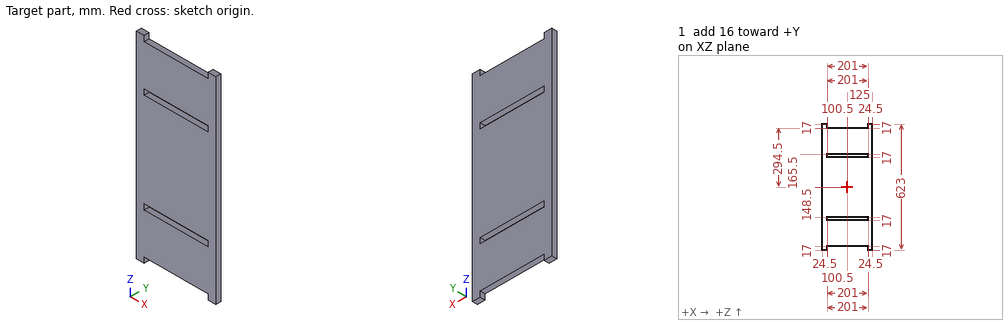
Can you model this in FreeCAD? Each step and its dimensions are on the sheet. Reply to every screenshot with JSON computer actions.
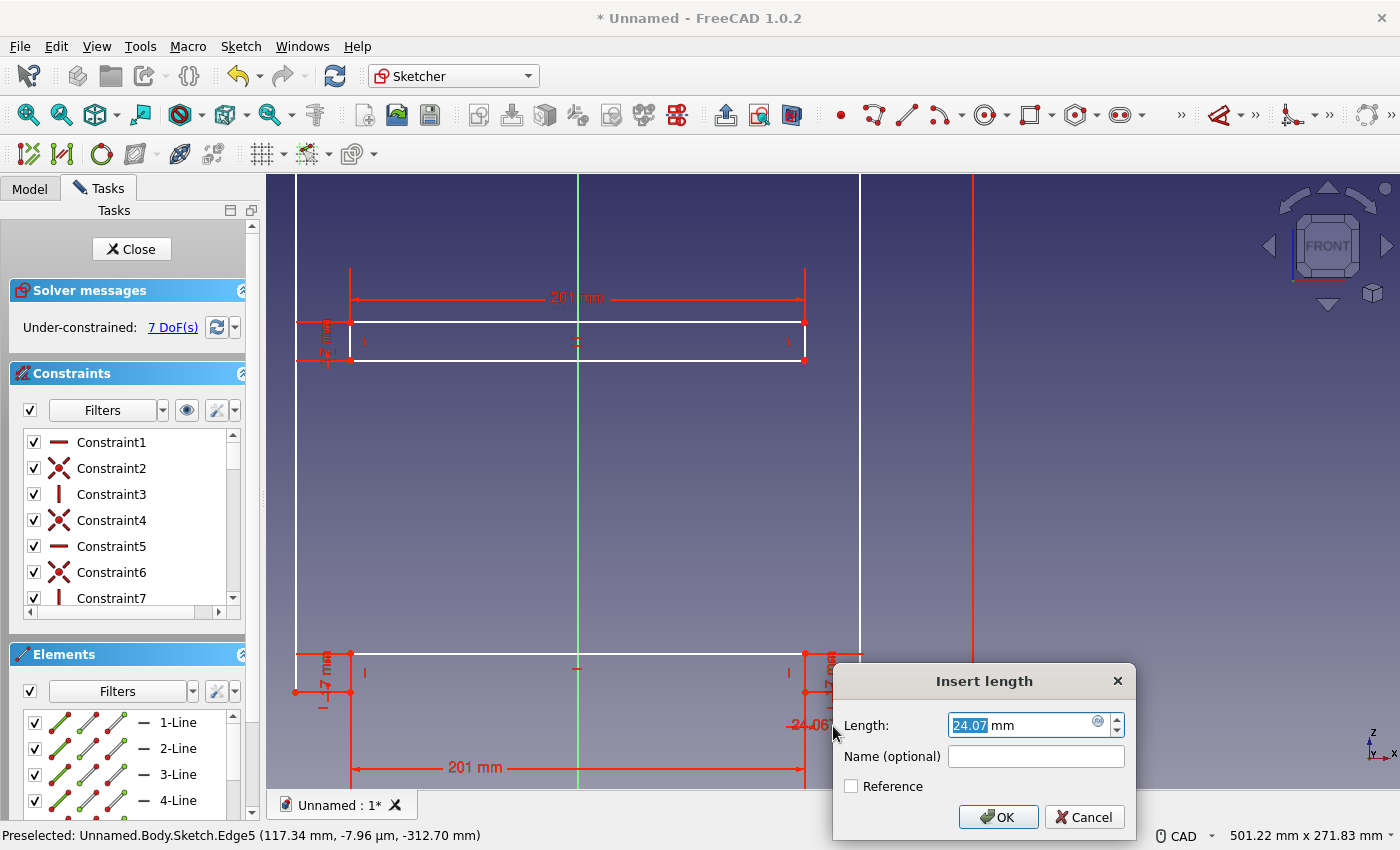
{"action": "type", "text": "24.5"}
{"action": "key", "text": "Return"}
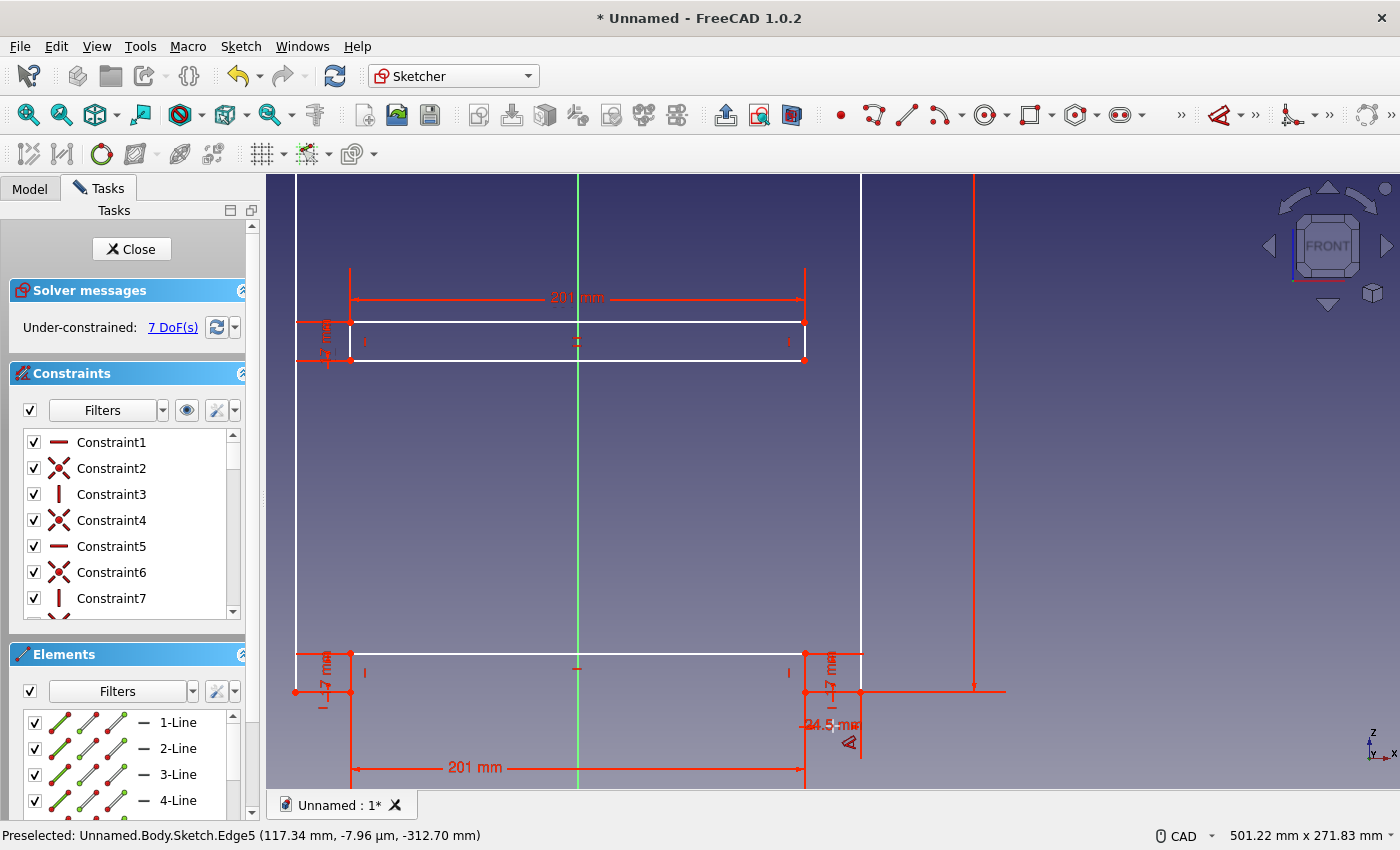
{"action": "left_click", "coordinate": [334, 692]}
{"action": "left_click", "coordinate": [323, 726]}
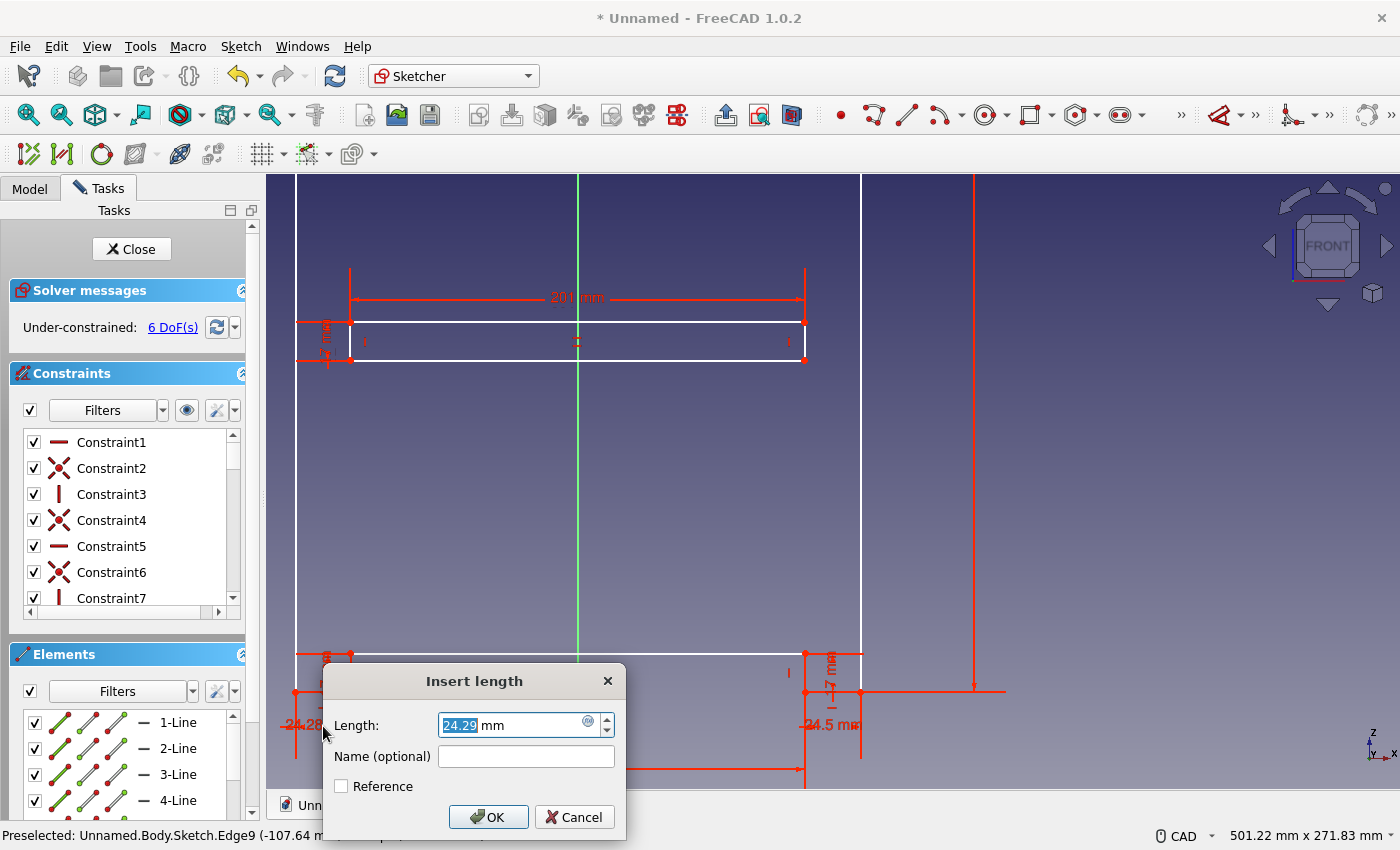
{"action": "type", "text": "24.5"}
{"action": "key", "text": "Return"}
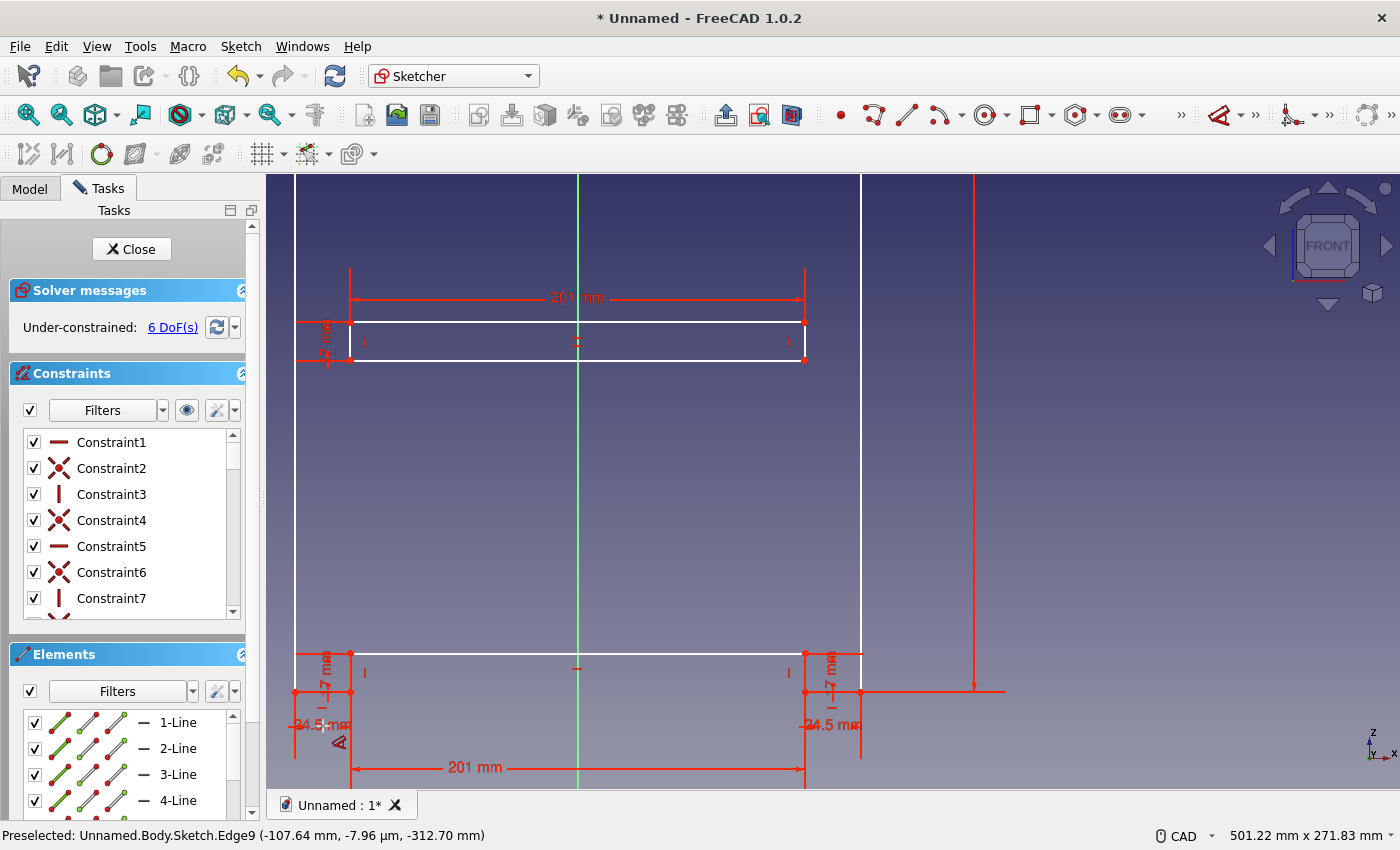
{"action": "scroll", "coordinate": [845, 696], "scroll_direction": "down", "scroll_amount": 6}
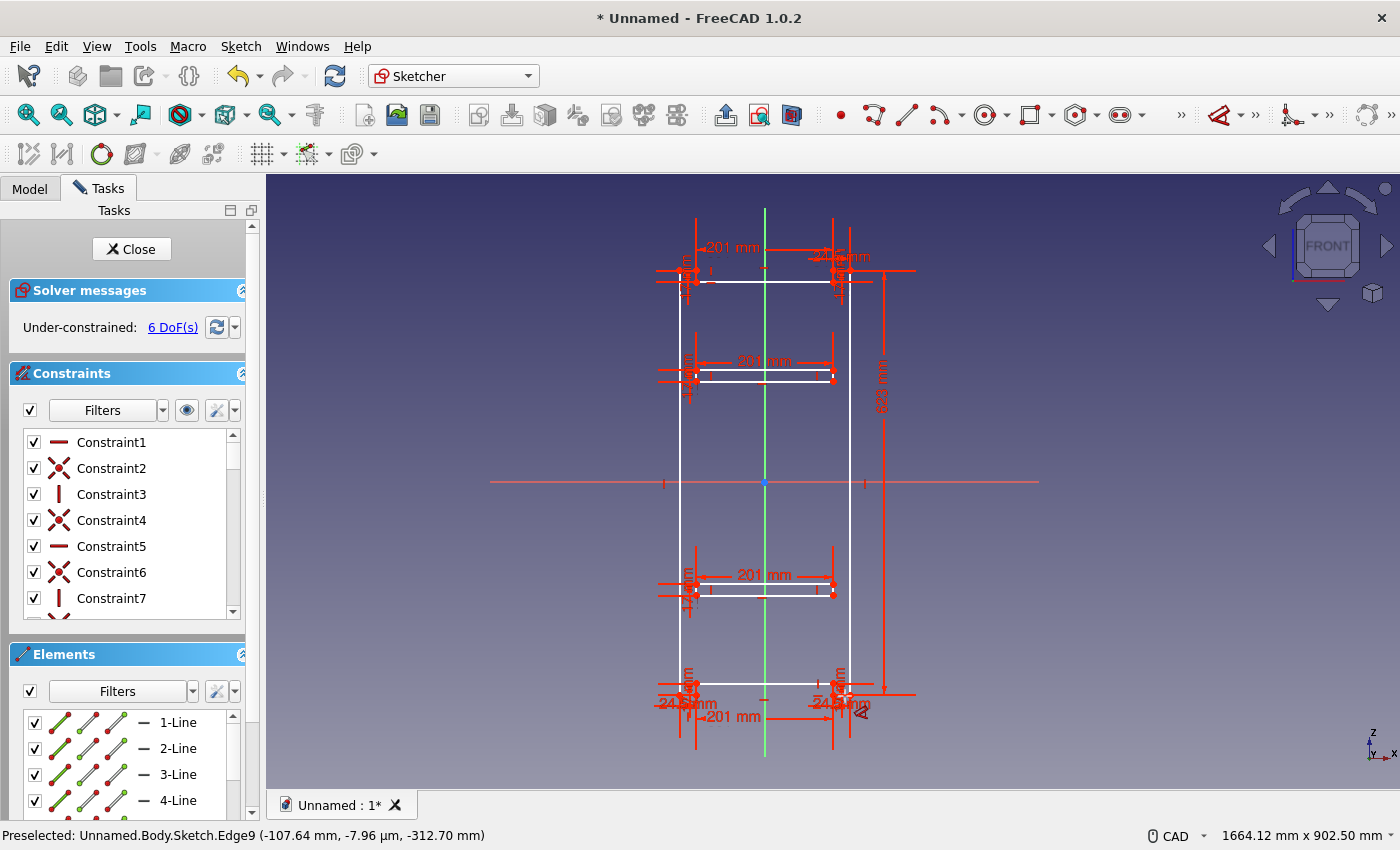
{"action": "left_click", "coordinate": [850, 271]}
{"action": "left_click", "coordinate": [807, 237]}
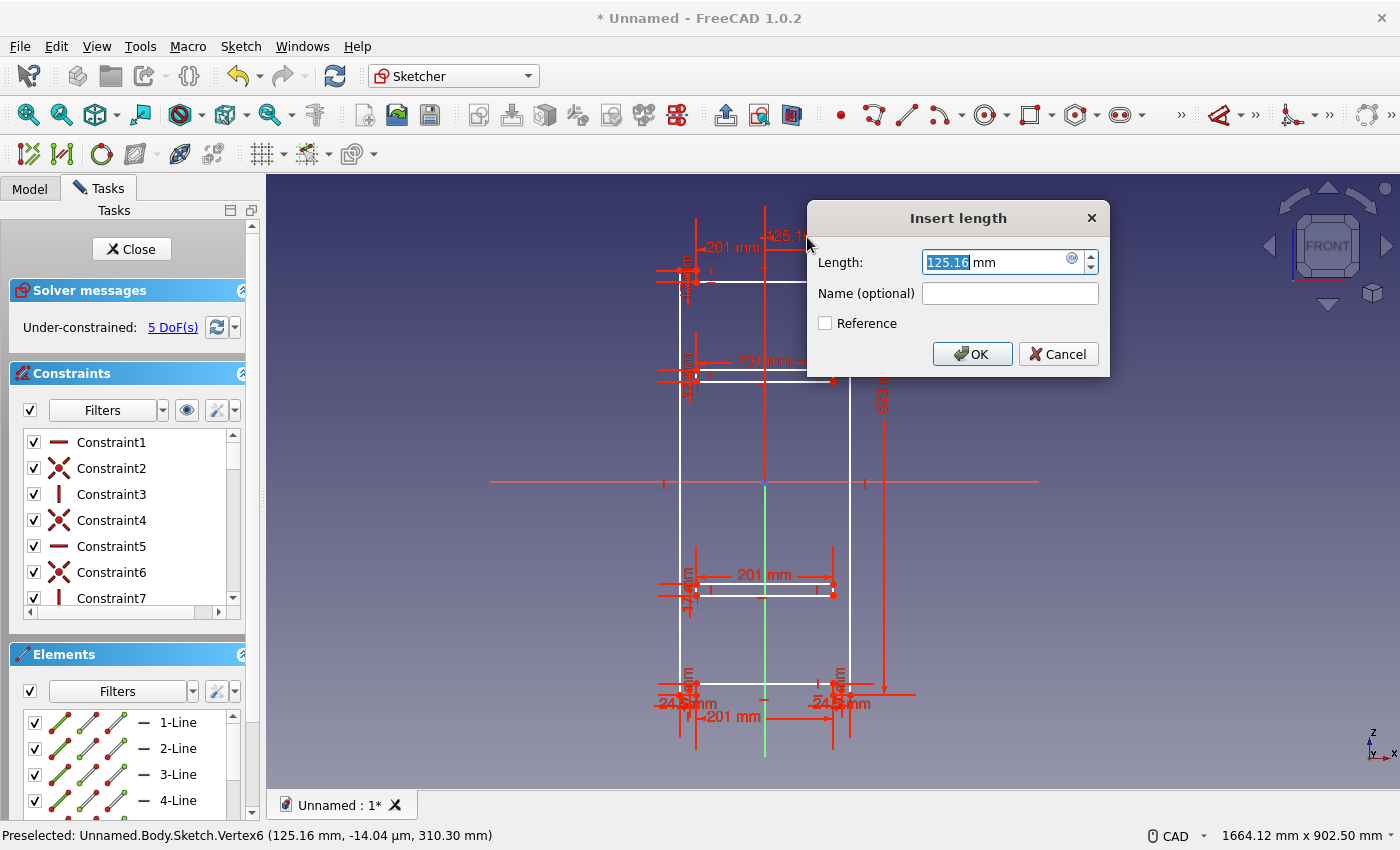
{"action": "type", "text": "125"}
{"action": "key", "text": "Return"}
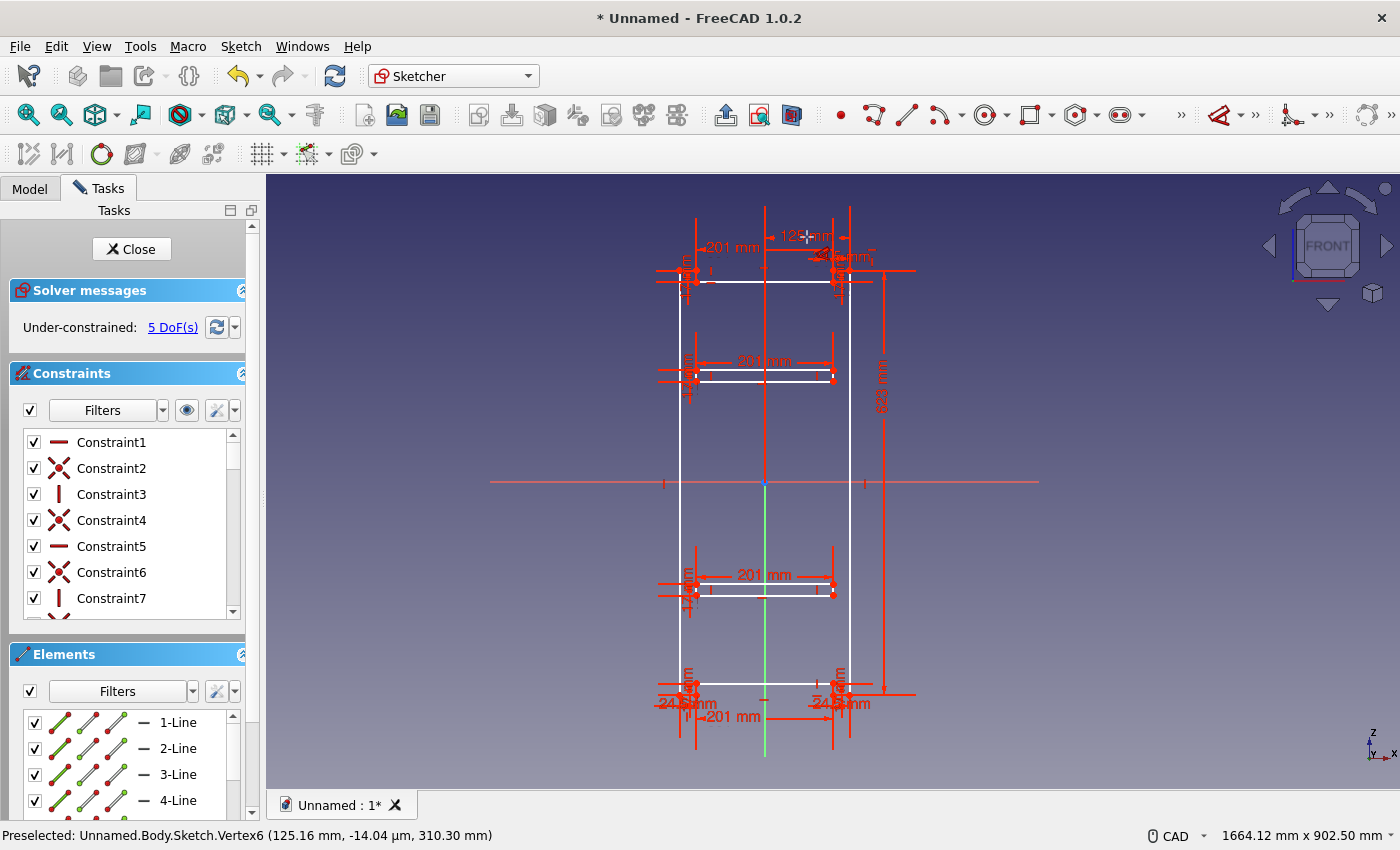
{"action": "left_click", "coordinate": [696, 282]}
{"action": "left_click", "coordinate": [662, 382]}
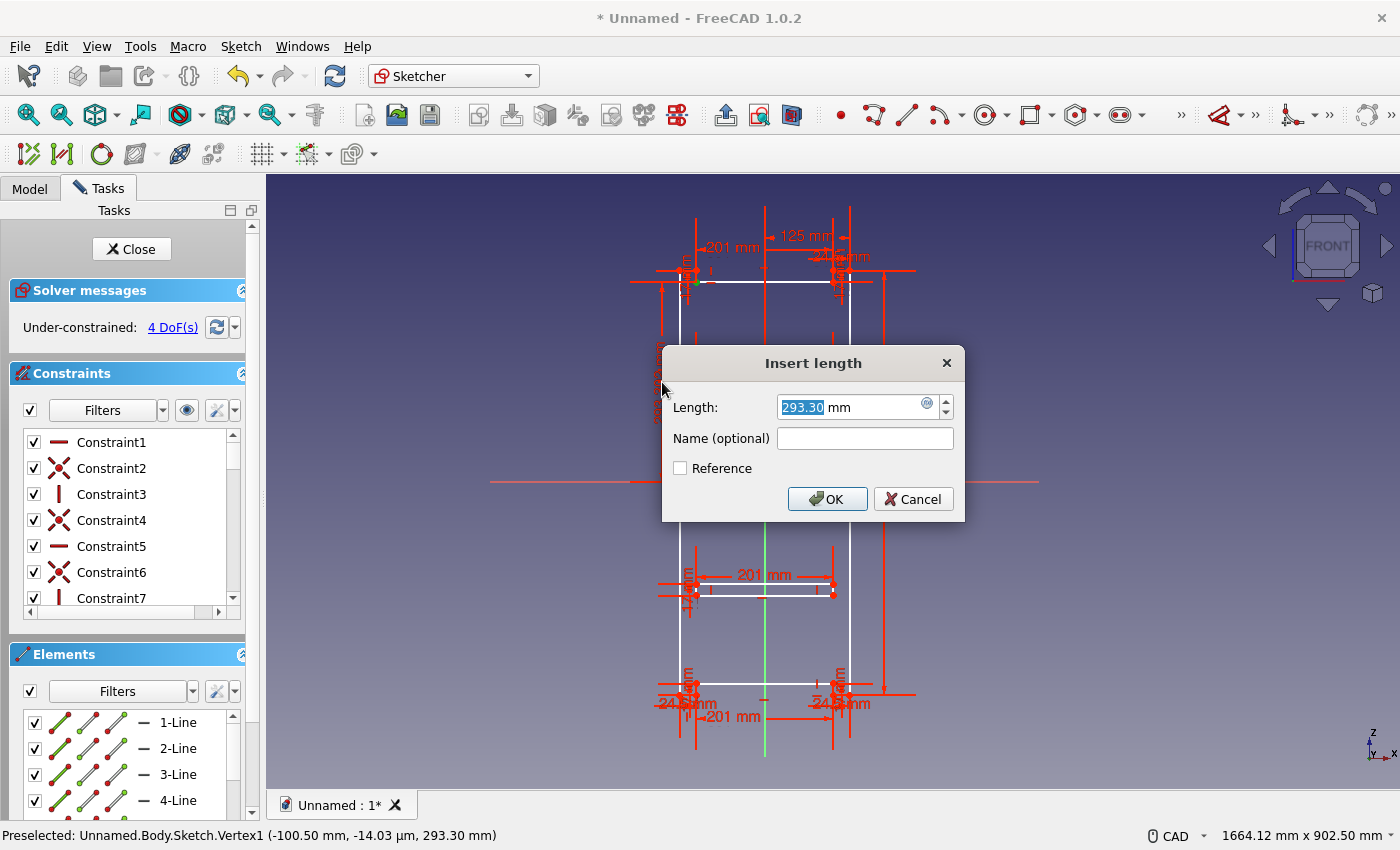
{"action": "type", "text": "294.5"}
{"action": "key", "text": "Return"}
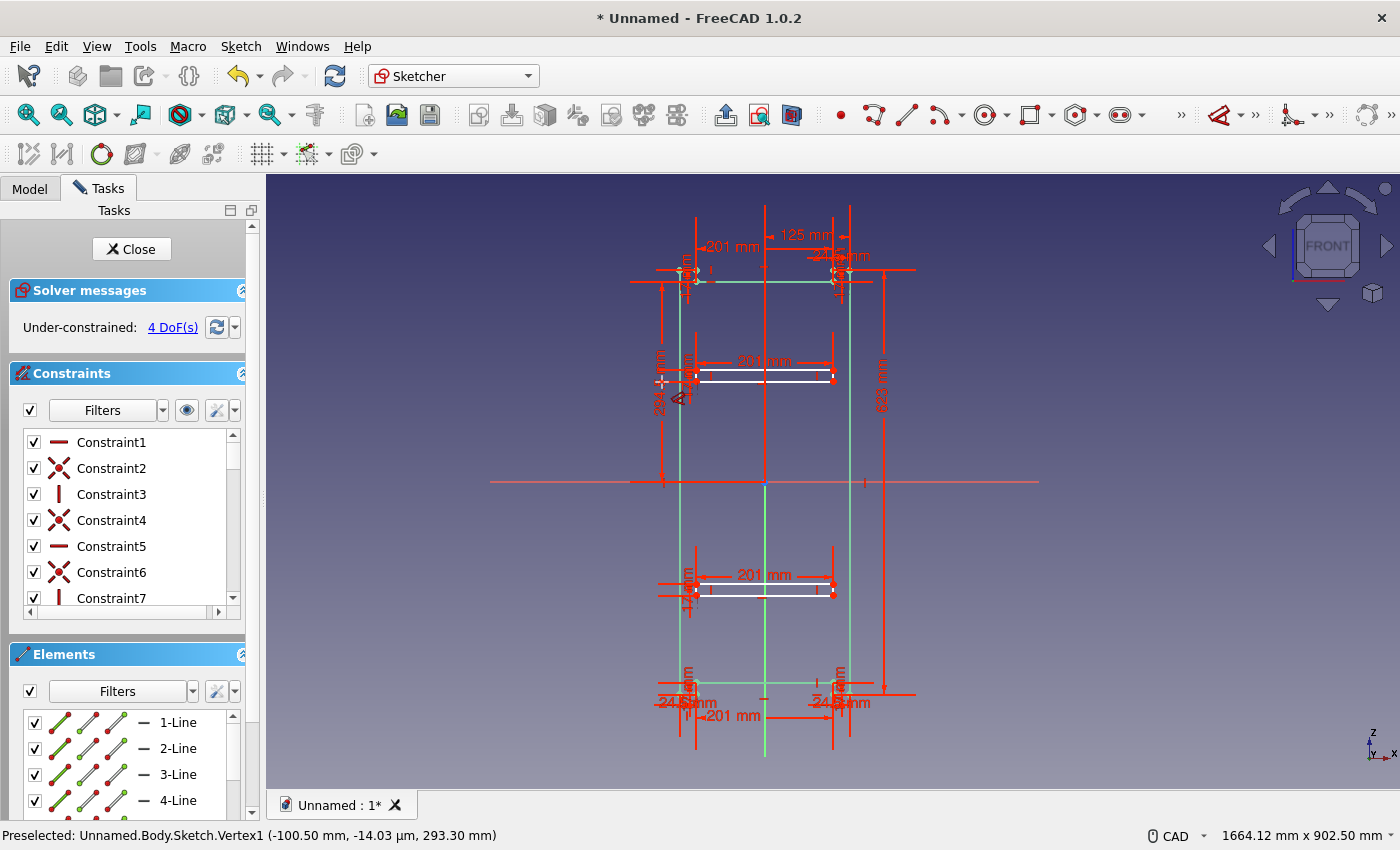
{"action": "left_click", "coordinate": [696, 370]}
{"action": "left_click", "coordinate": [731, 336]}